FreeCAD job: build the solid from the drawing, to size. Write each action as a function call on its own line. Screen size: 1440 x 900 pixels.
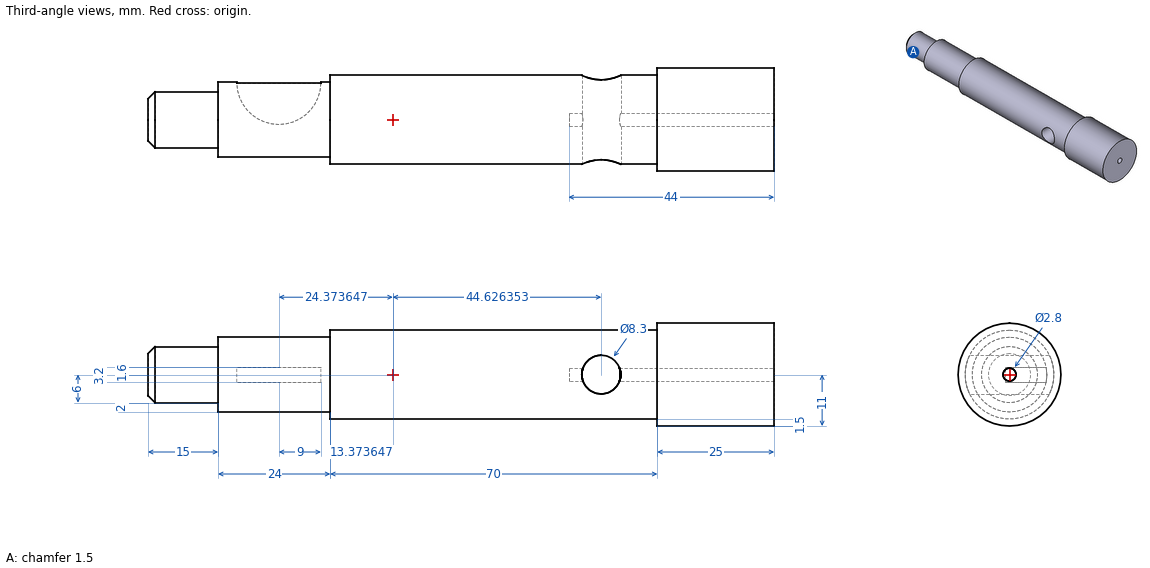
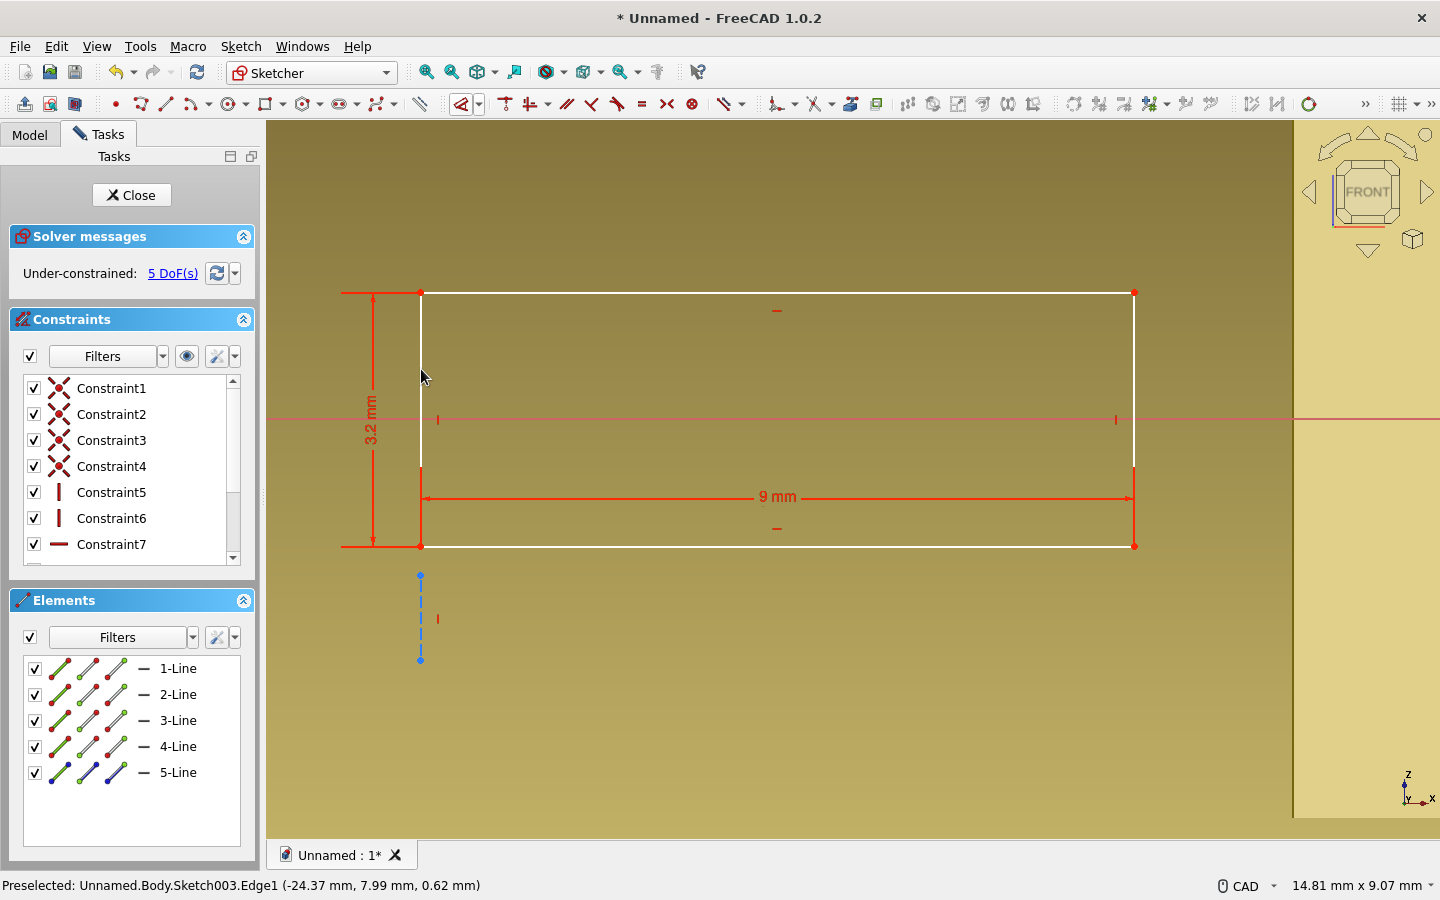
click(421, 293)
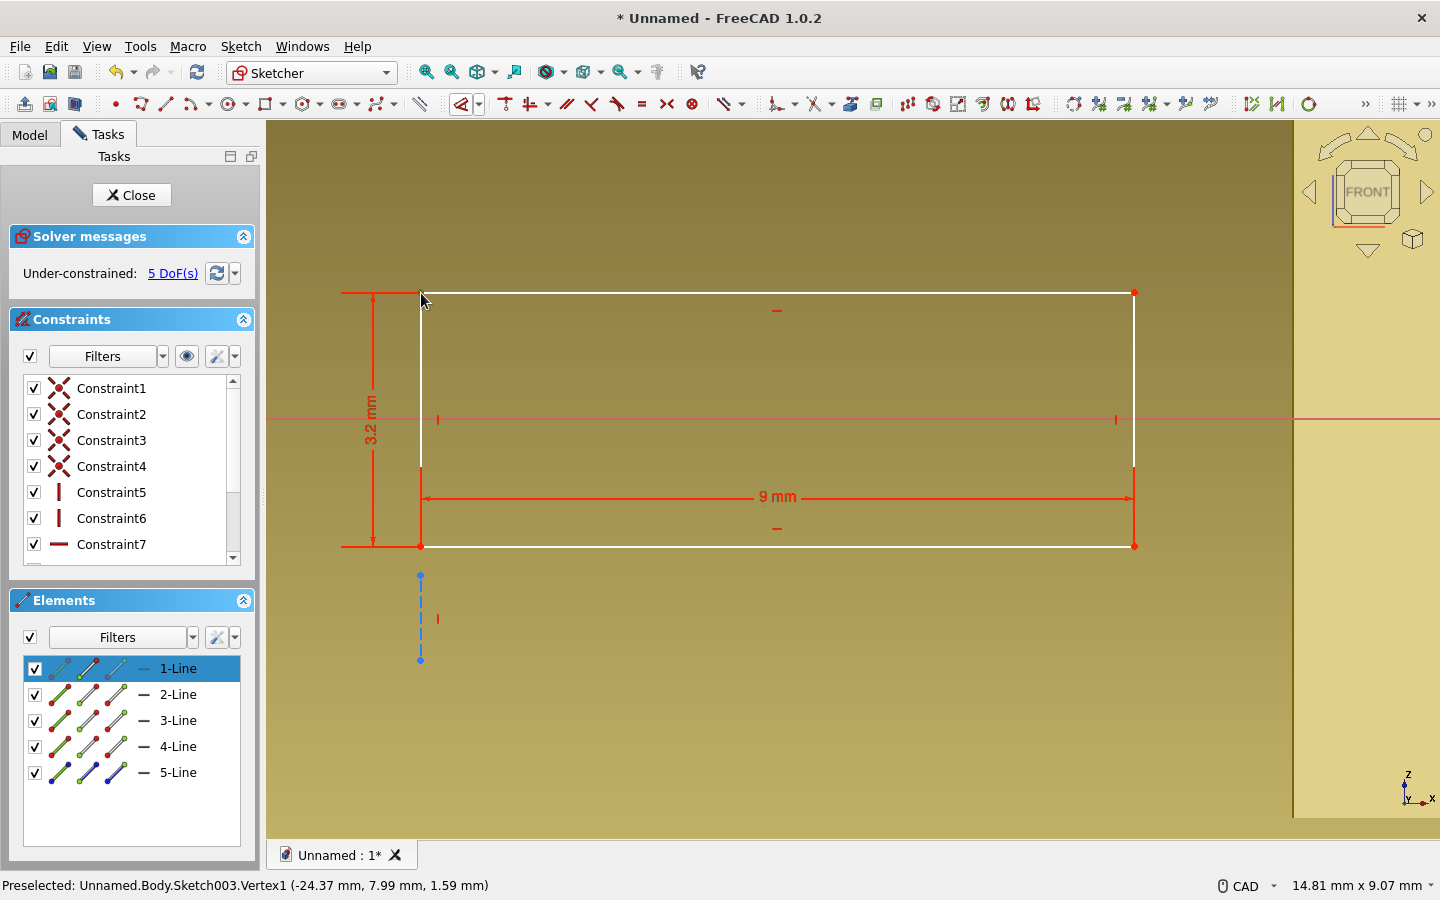
key(i)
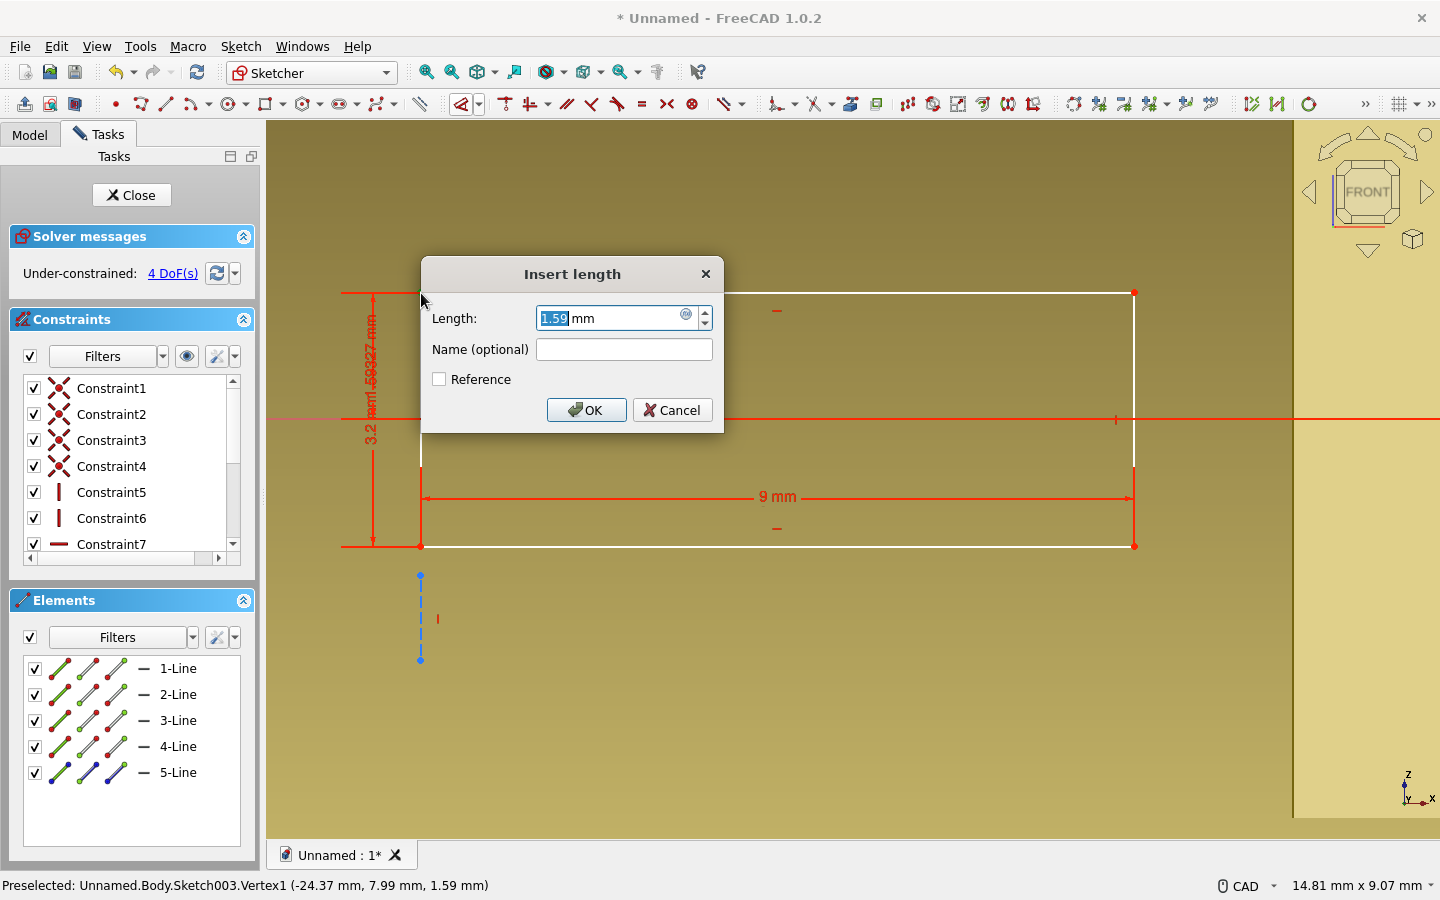
text(1.6)
key(Return)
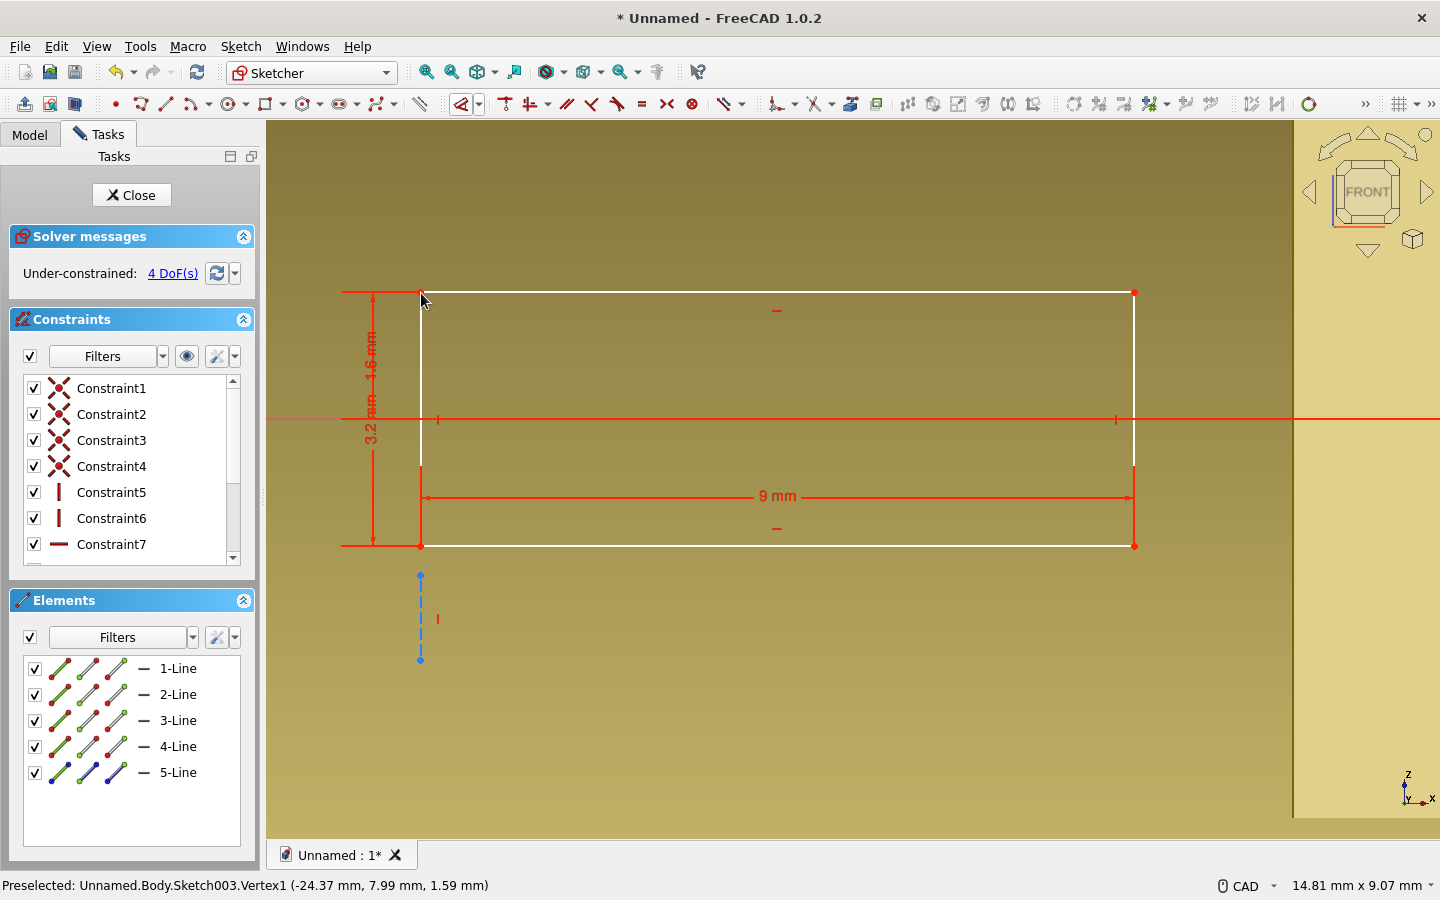
click(421, 292)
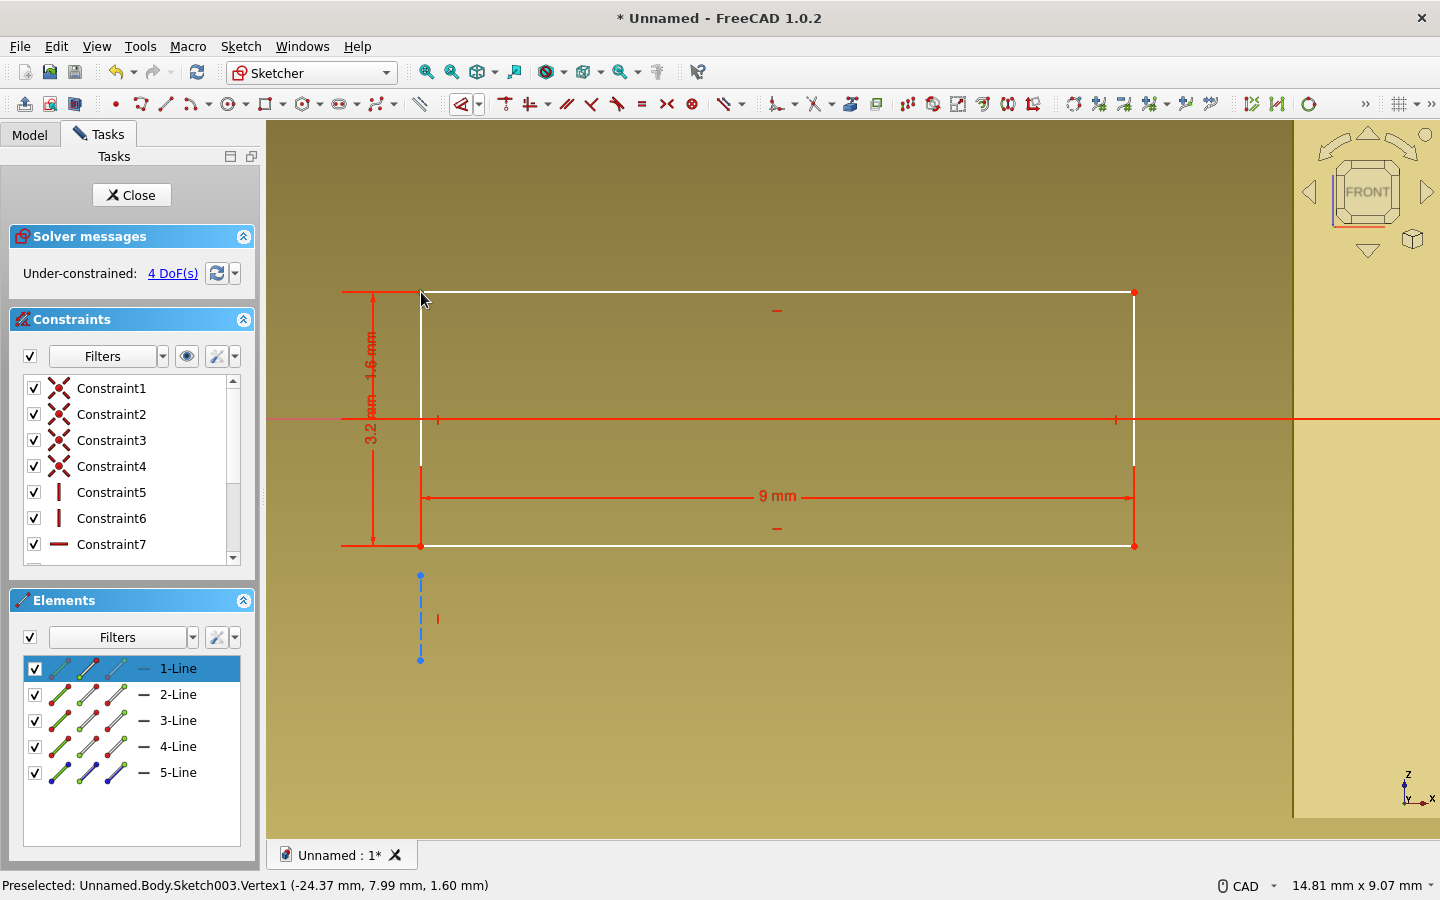
click(478, 104)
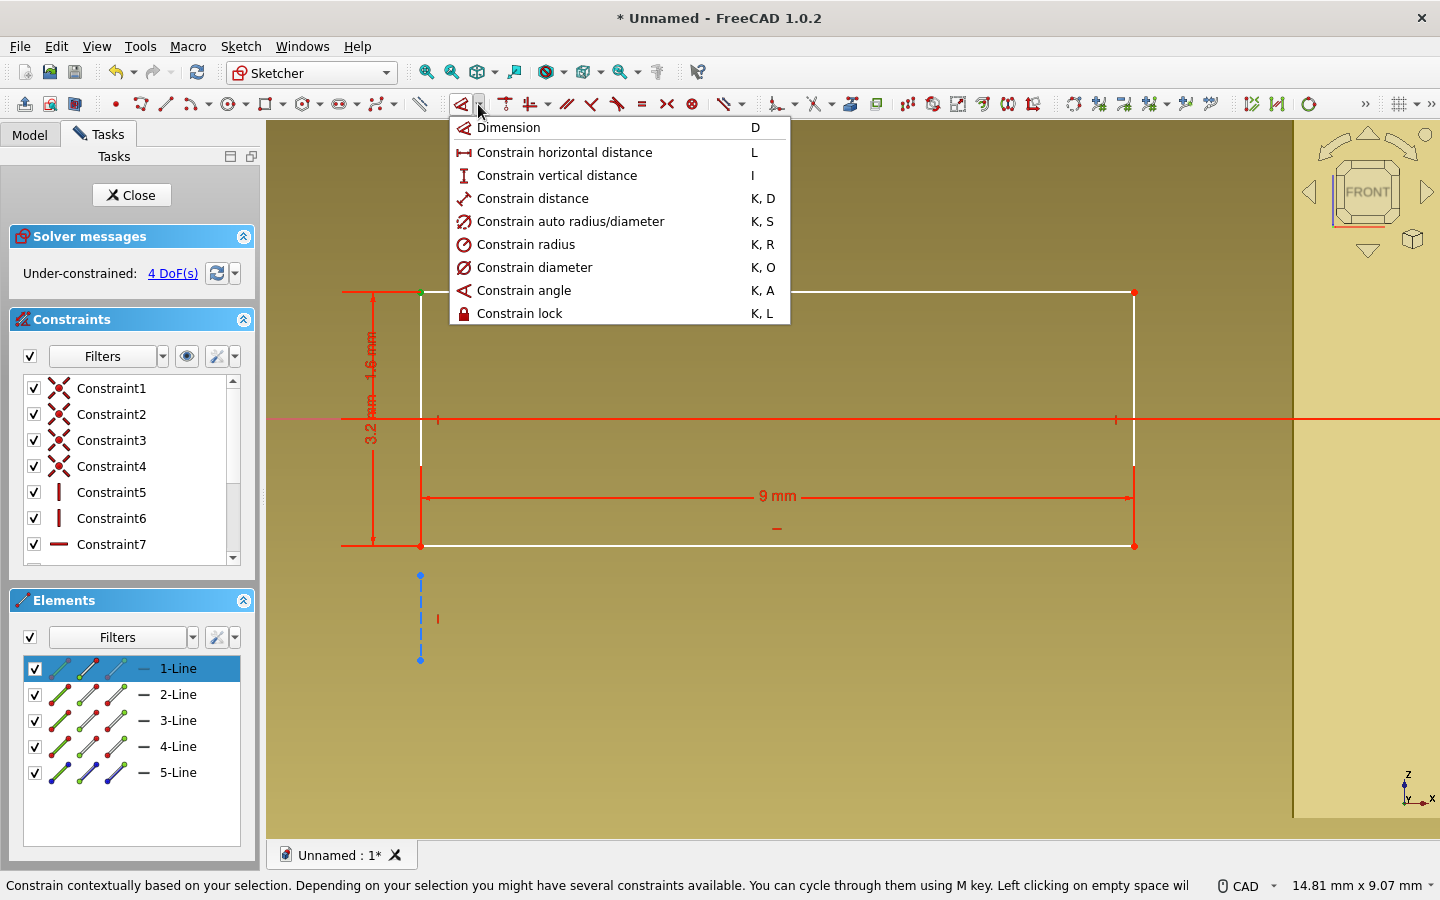
click(620, 152)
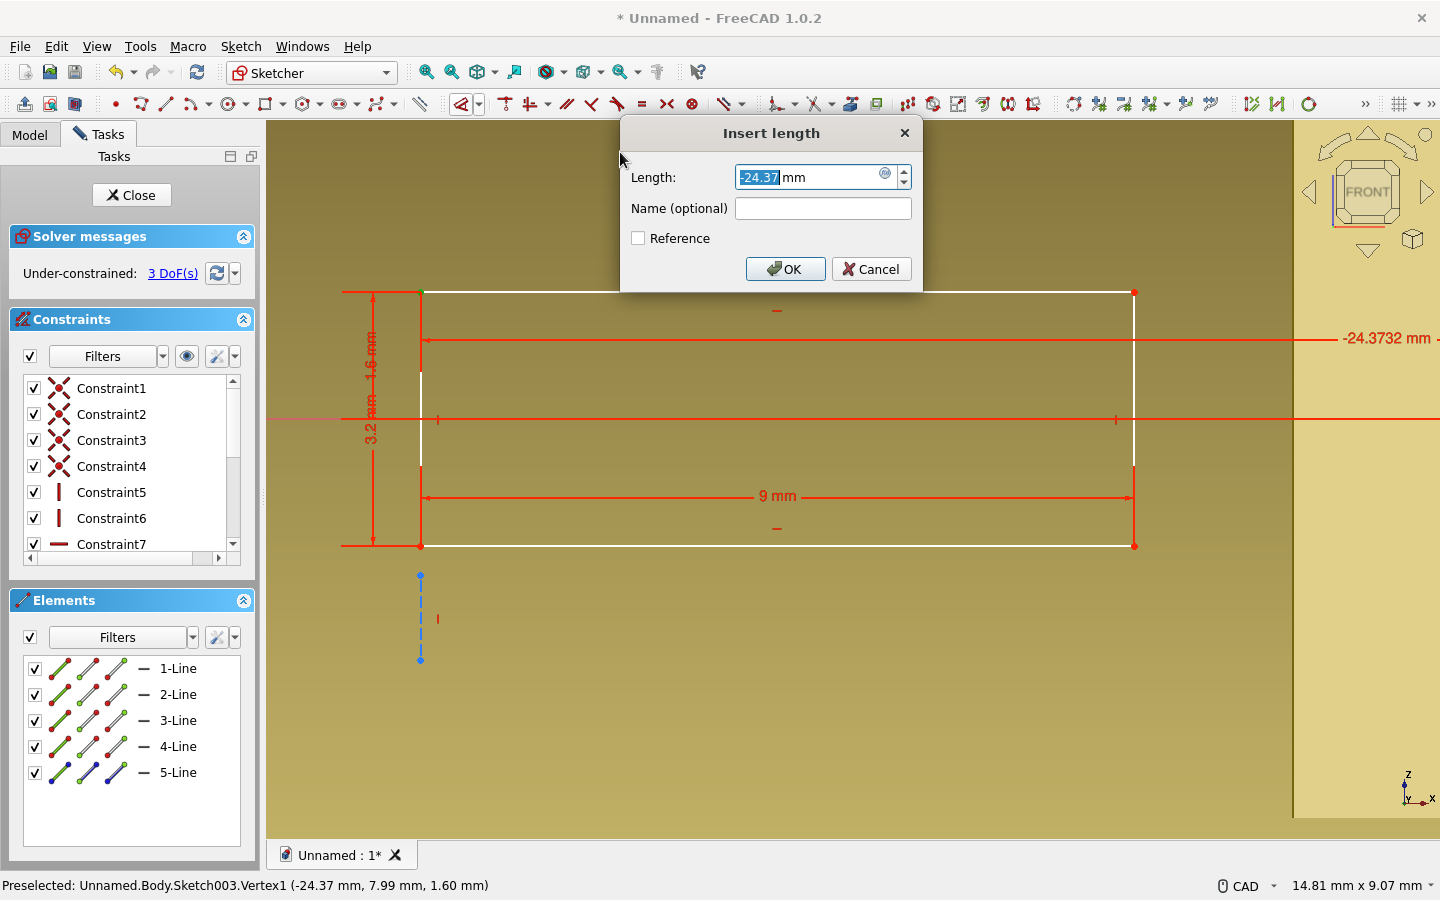
text(-24.373647)
key(Return)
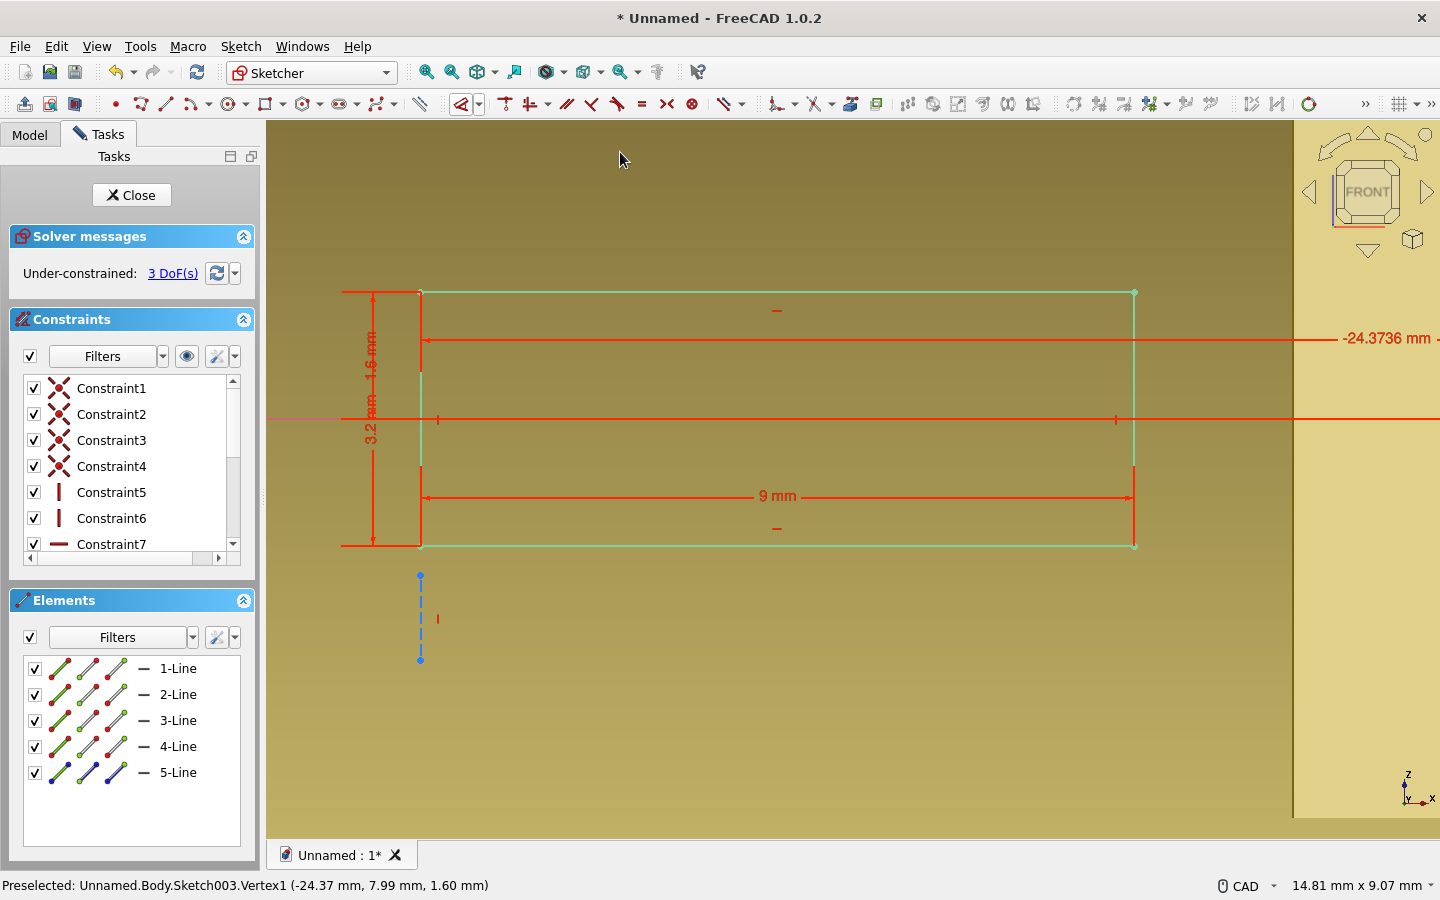
click(421, 576)